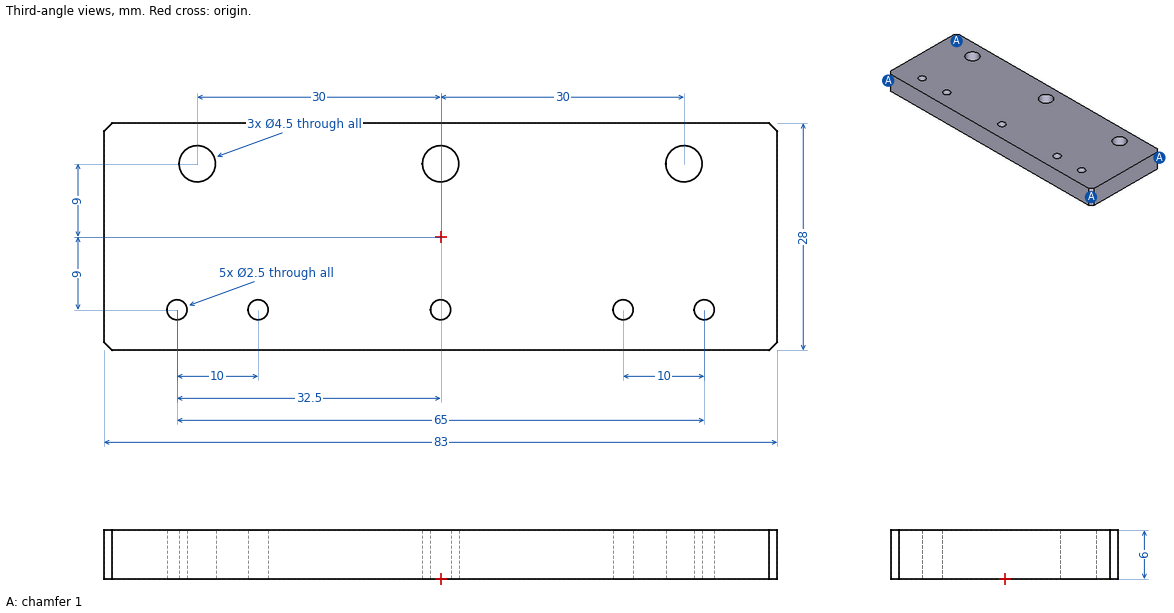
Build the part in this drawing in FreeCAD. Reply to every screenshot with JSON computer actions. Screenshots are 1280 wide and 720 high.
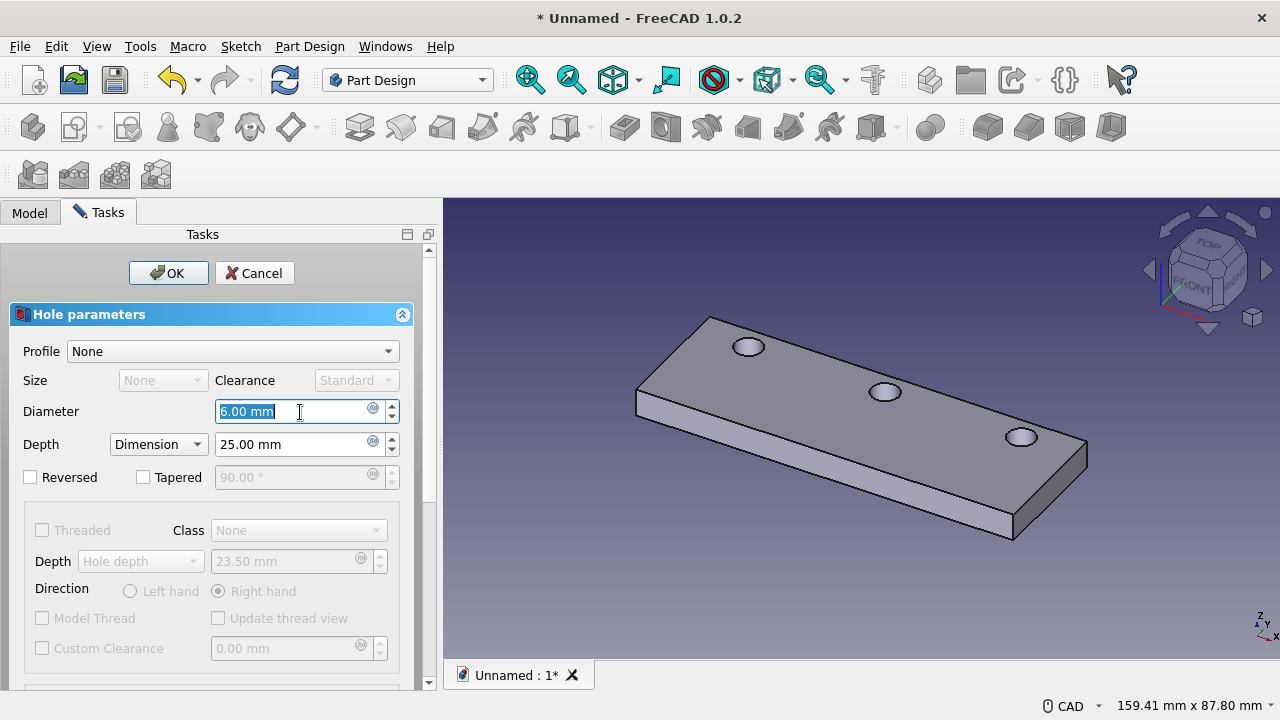
{"action": "type", "text": "4.5"}
{"action": "key", "text": "Tab"}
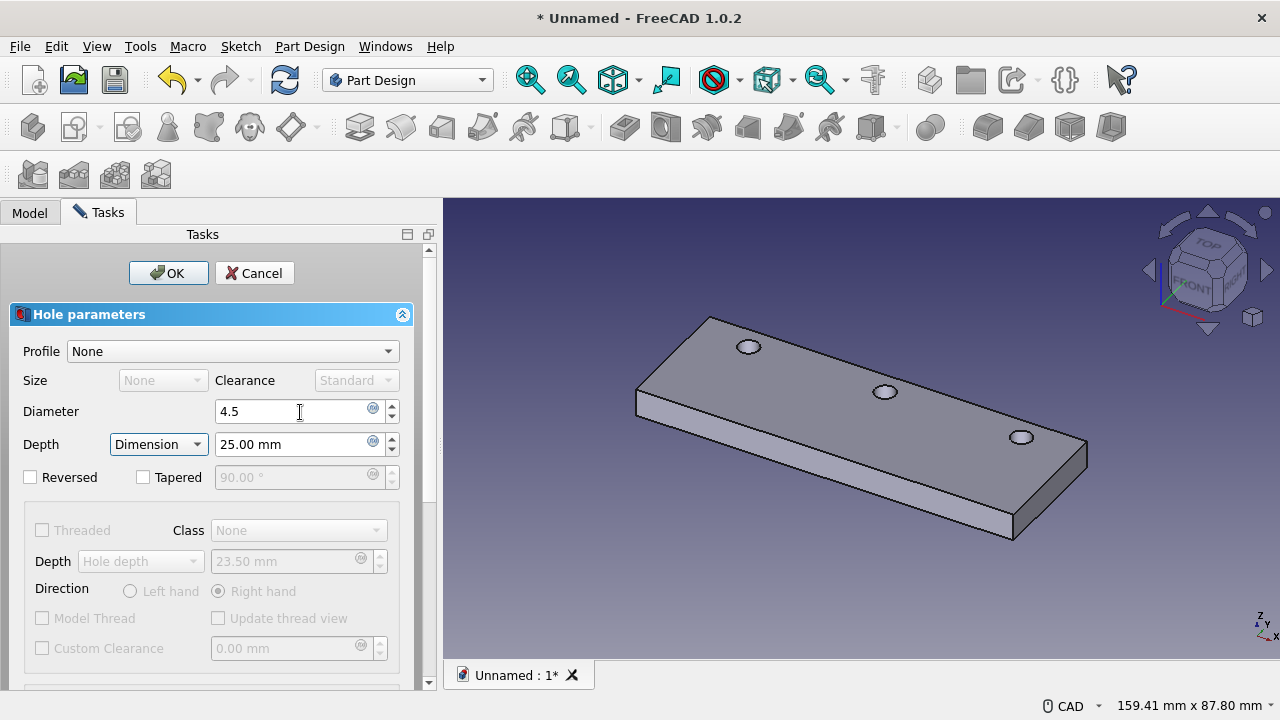
{"action": "left_click", "coordinate": [160, 444]}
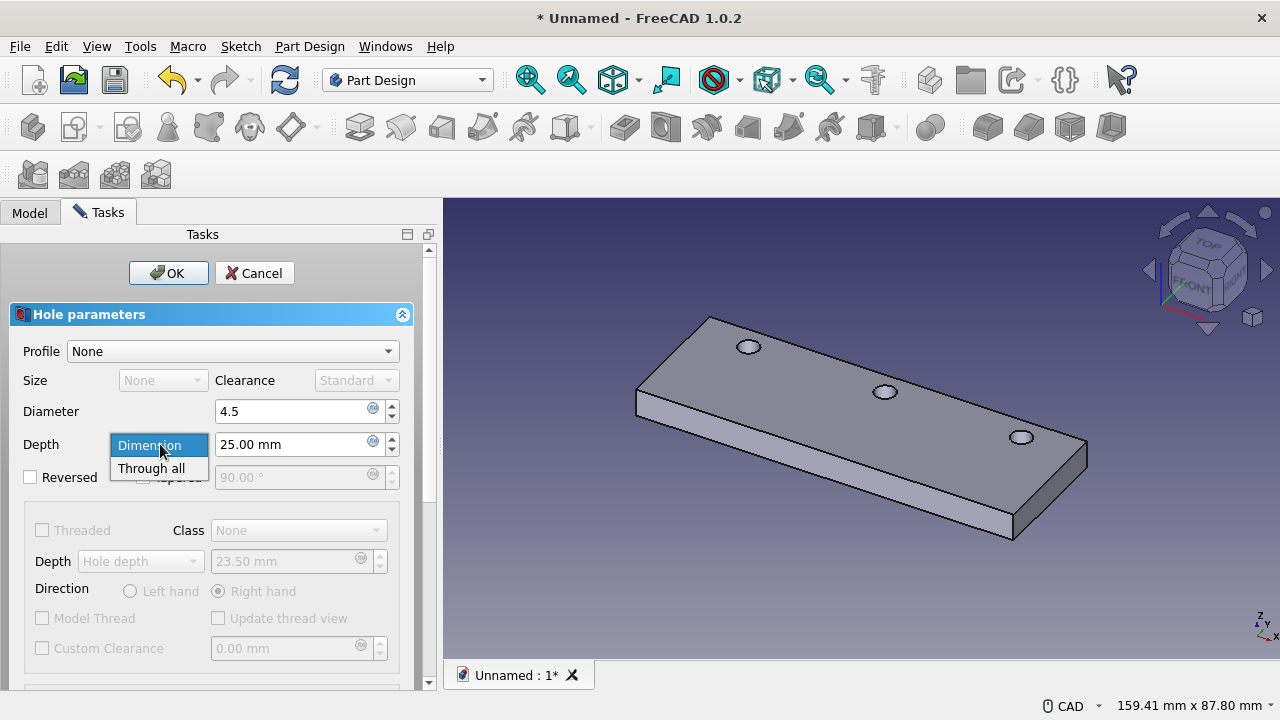
{"action": "left_click", "coordinate": [158, 468]}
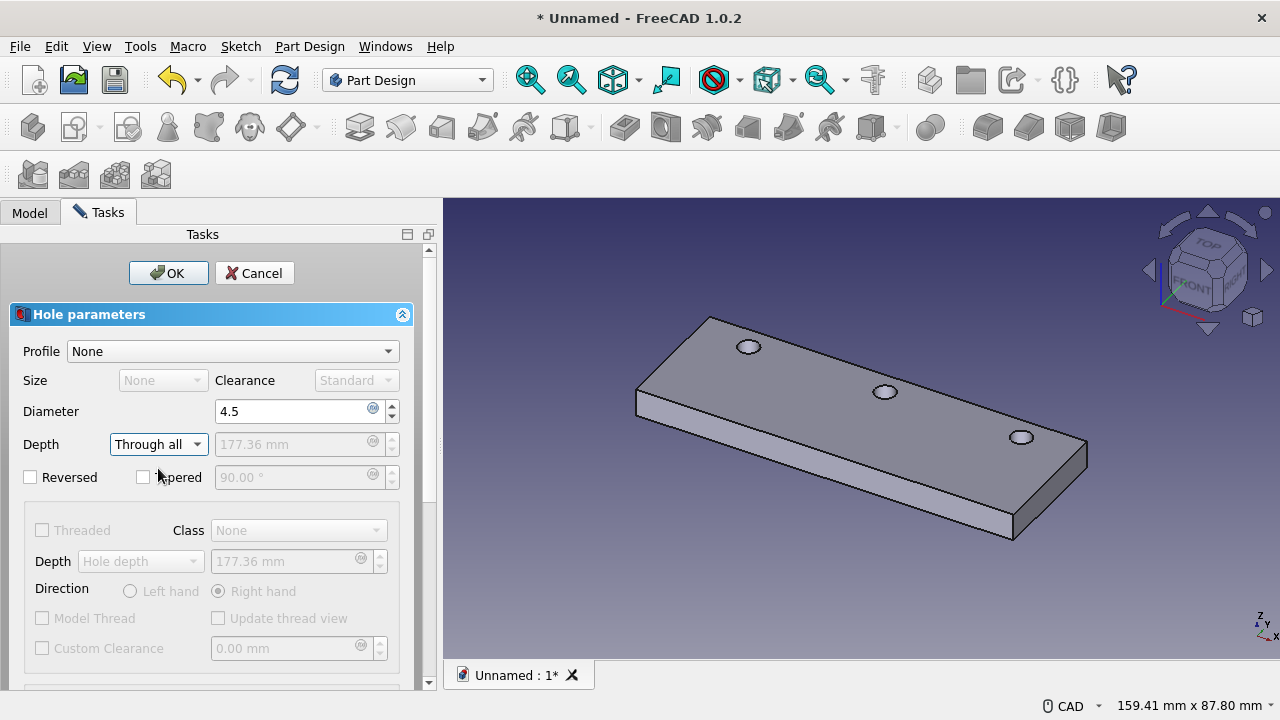
{"action": "left_click", "coordinate": [169, 273]}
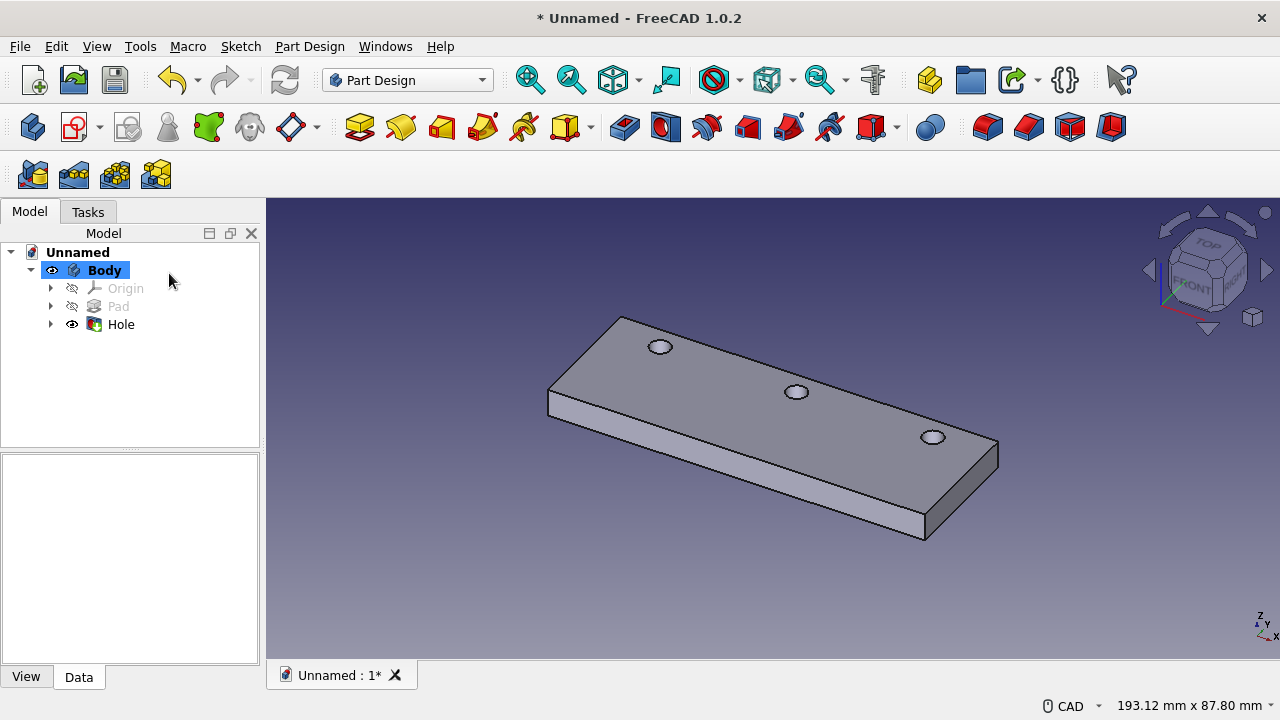
{"action": "left_click", "coordinate": [719, 397]}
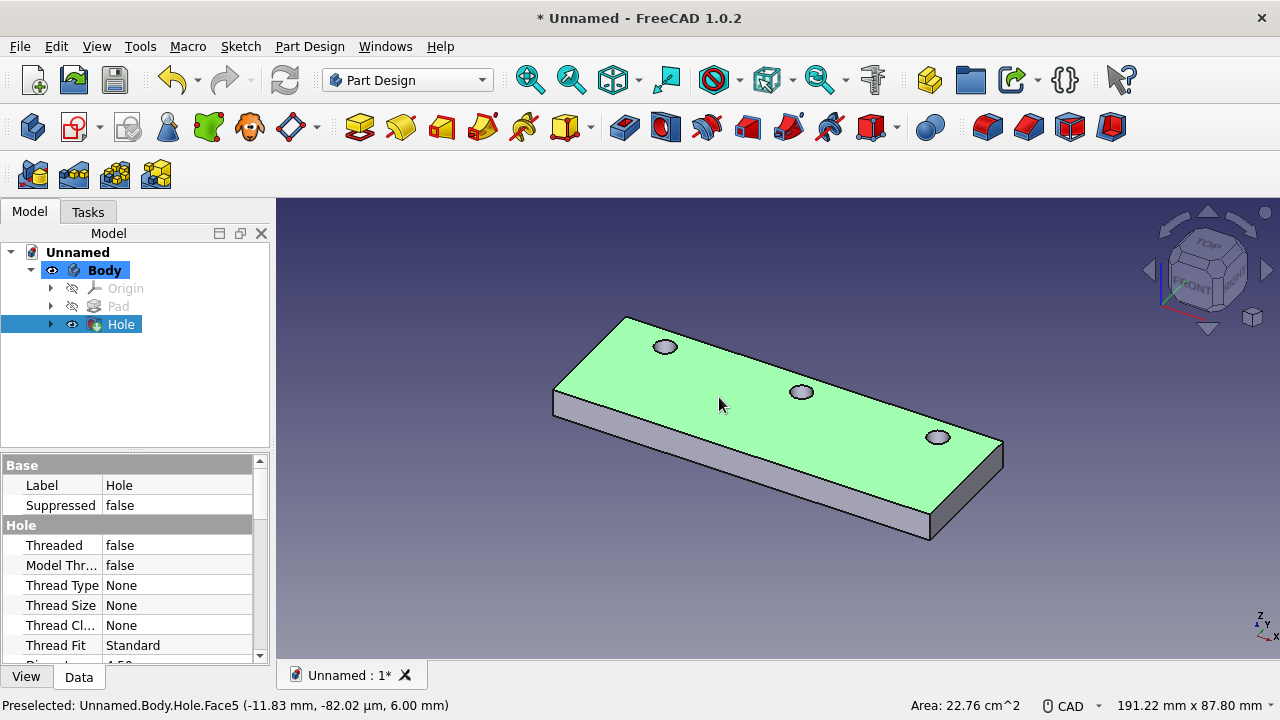
{"action": "left_click", "coordinate": [74, 128]}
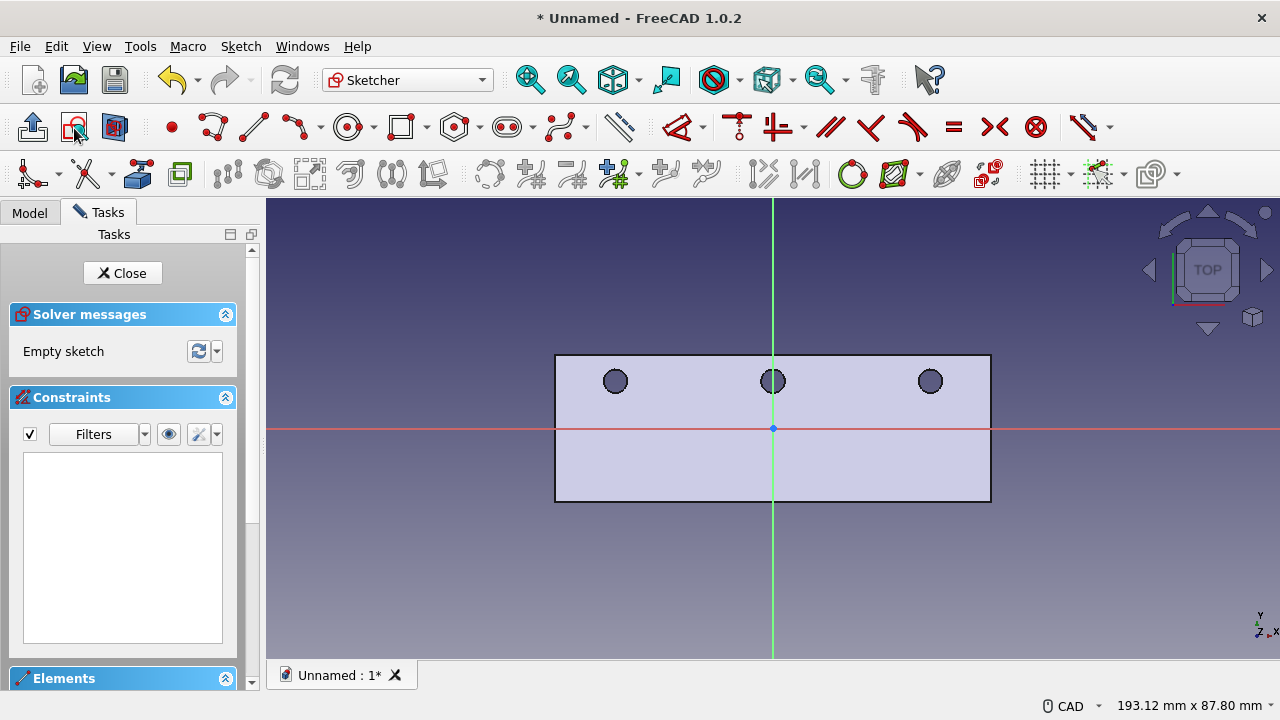
{"action": "scroll", "coordinate": [912, 510], "scroll_direction": "up", "scroll_amount": 2}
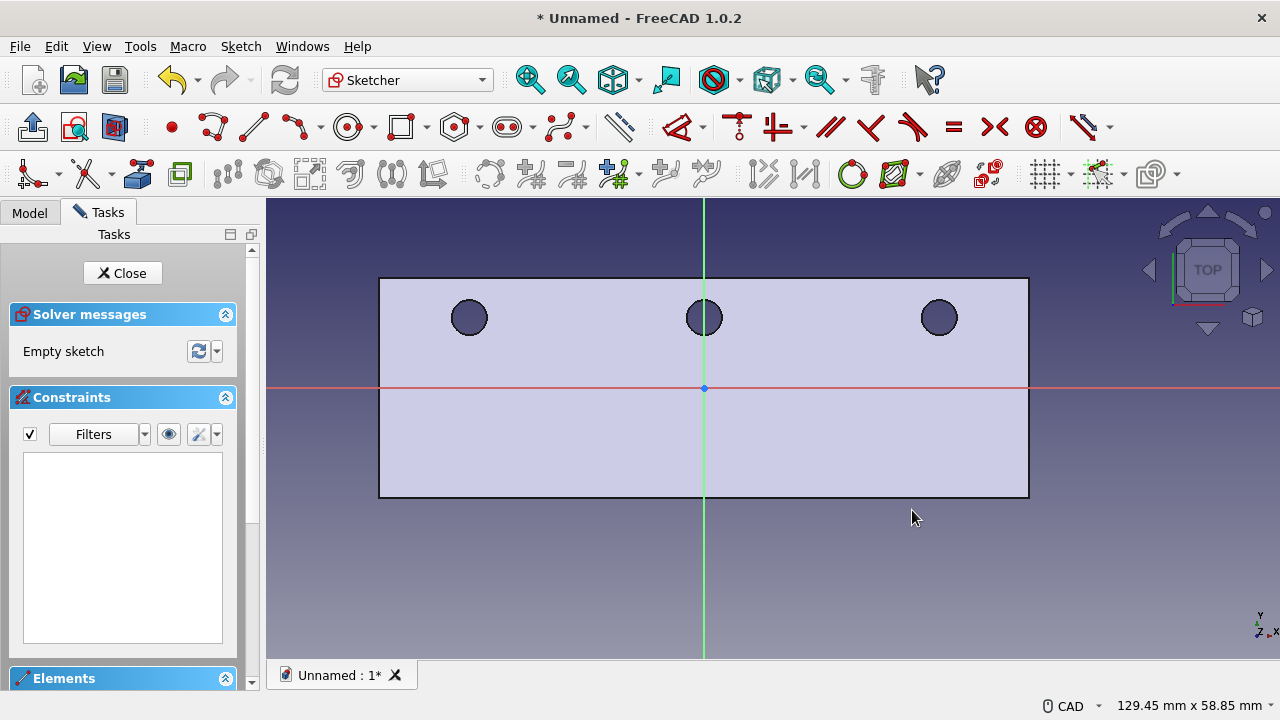
{"action": "left_click", "coordinate": [348, 128]}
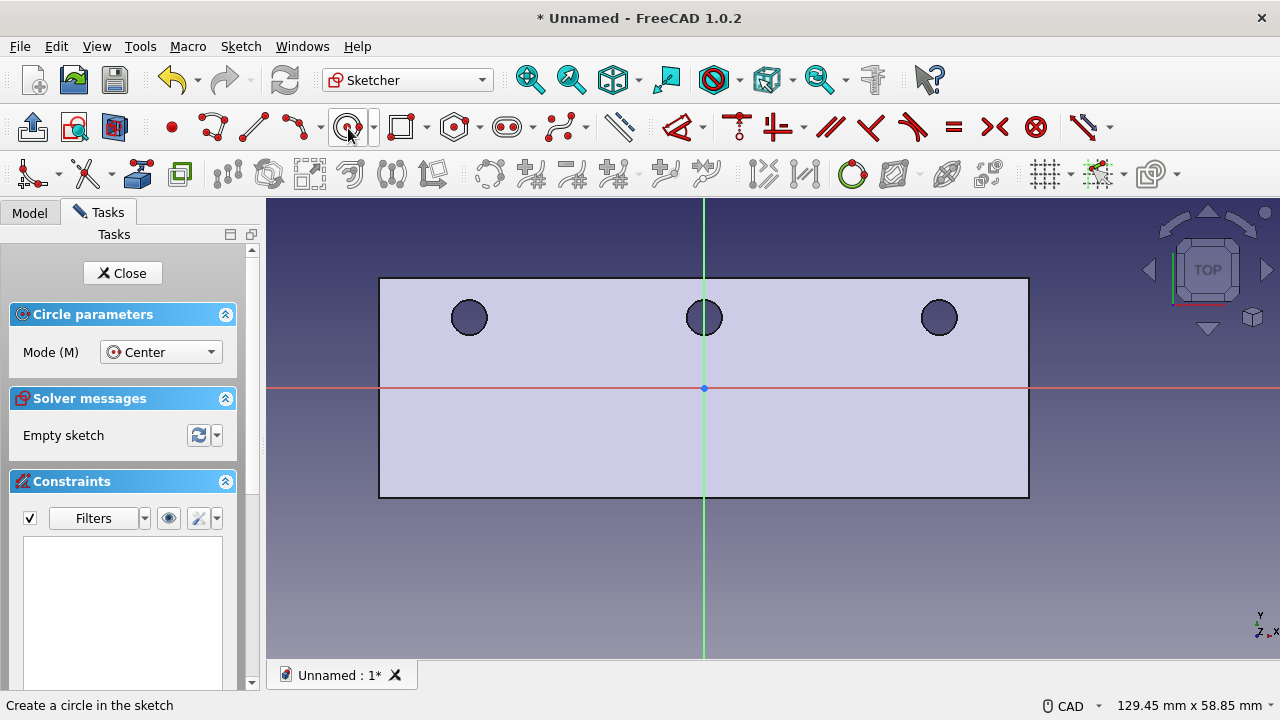
{"action": "scroll", "coordinate": [450, 459], "scroll_direction": "up", "scroll_amount": 5}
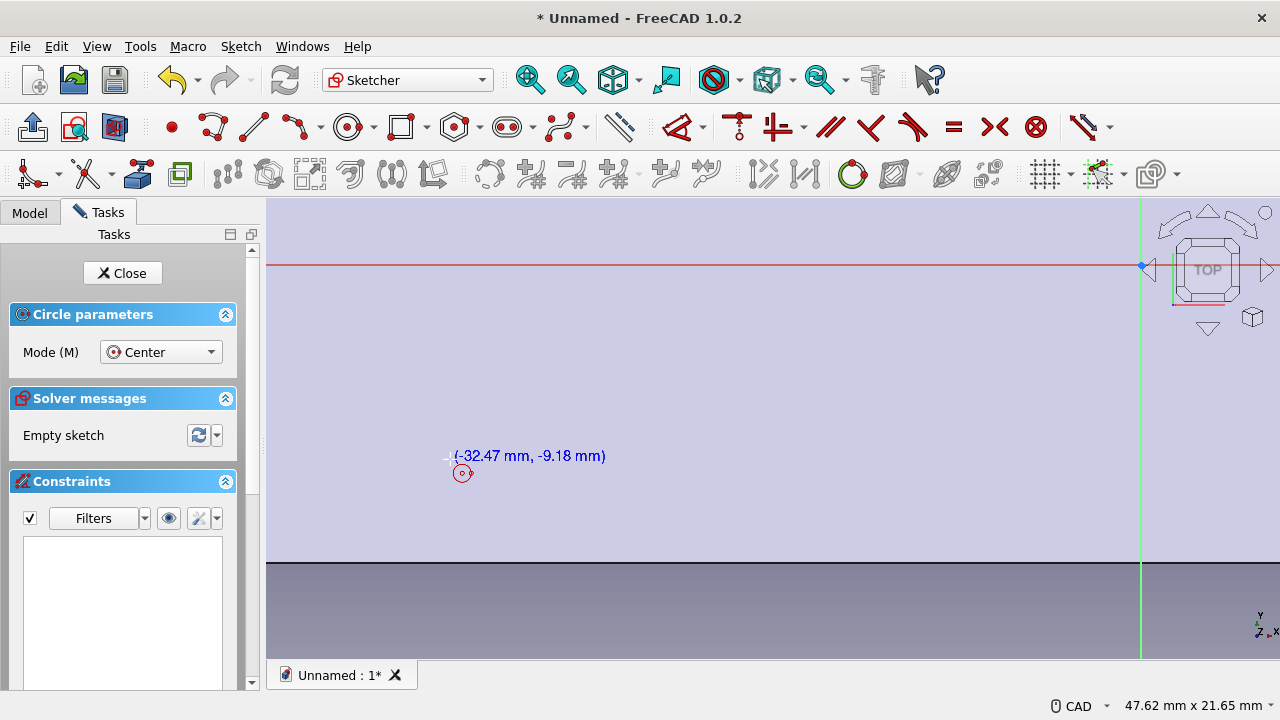
{"action": "left_click", "coordinate": [449, 457]}
{"action": "left_click", "coordinate": [468, 438]}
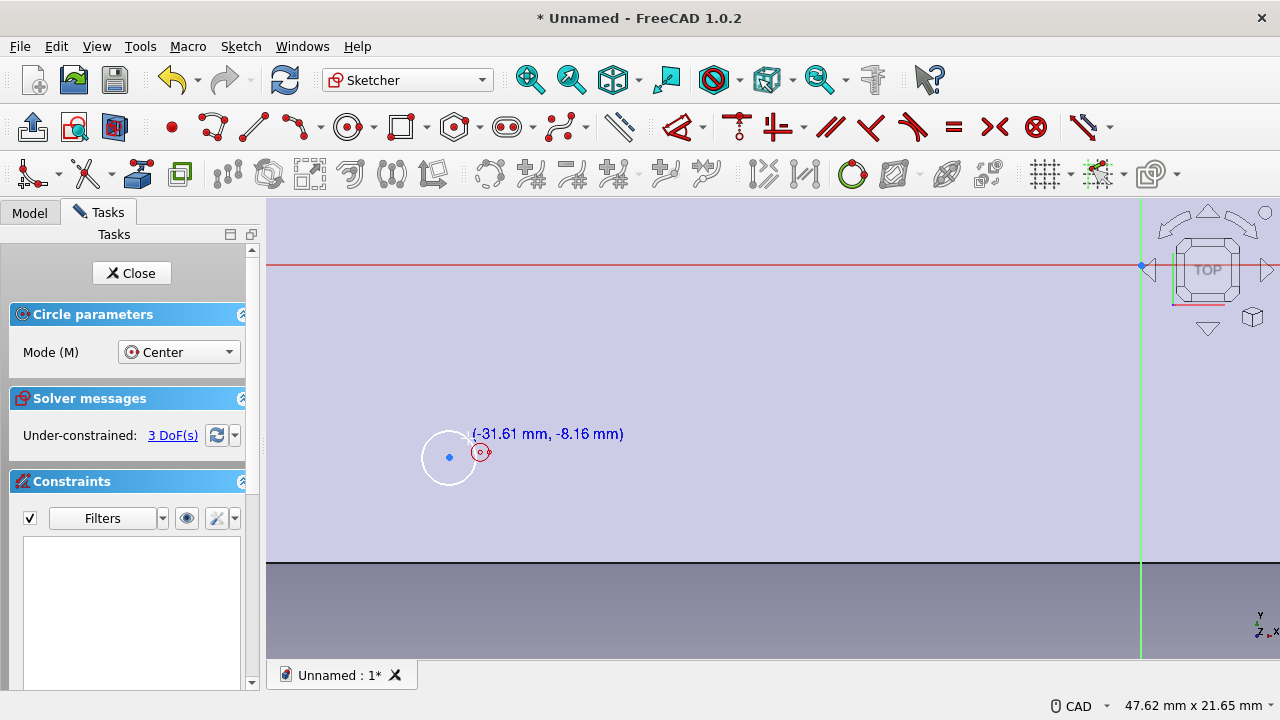
{"action": "scroll", "coordinate": [450, 460], "scroll_direction": "down", "scroll_amount": 5}